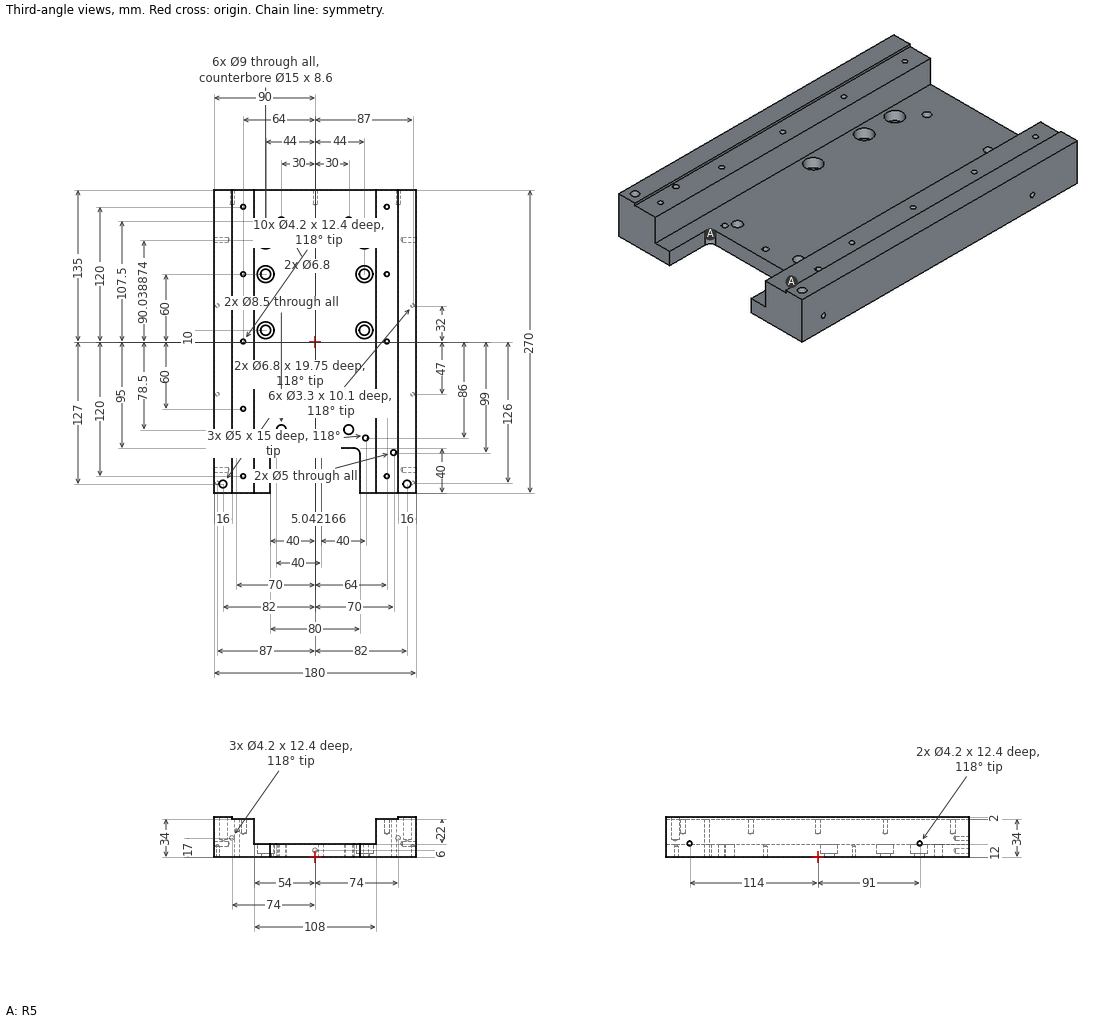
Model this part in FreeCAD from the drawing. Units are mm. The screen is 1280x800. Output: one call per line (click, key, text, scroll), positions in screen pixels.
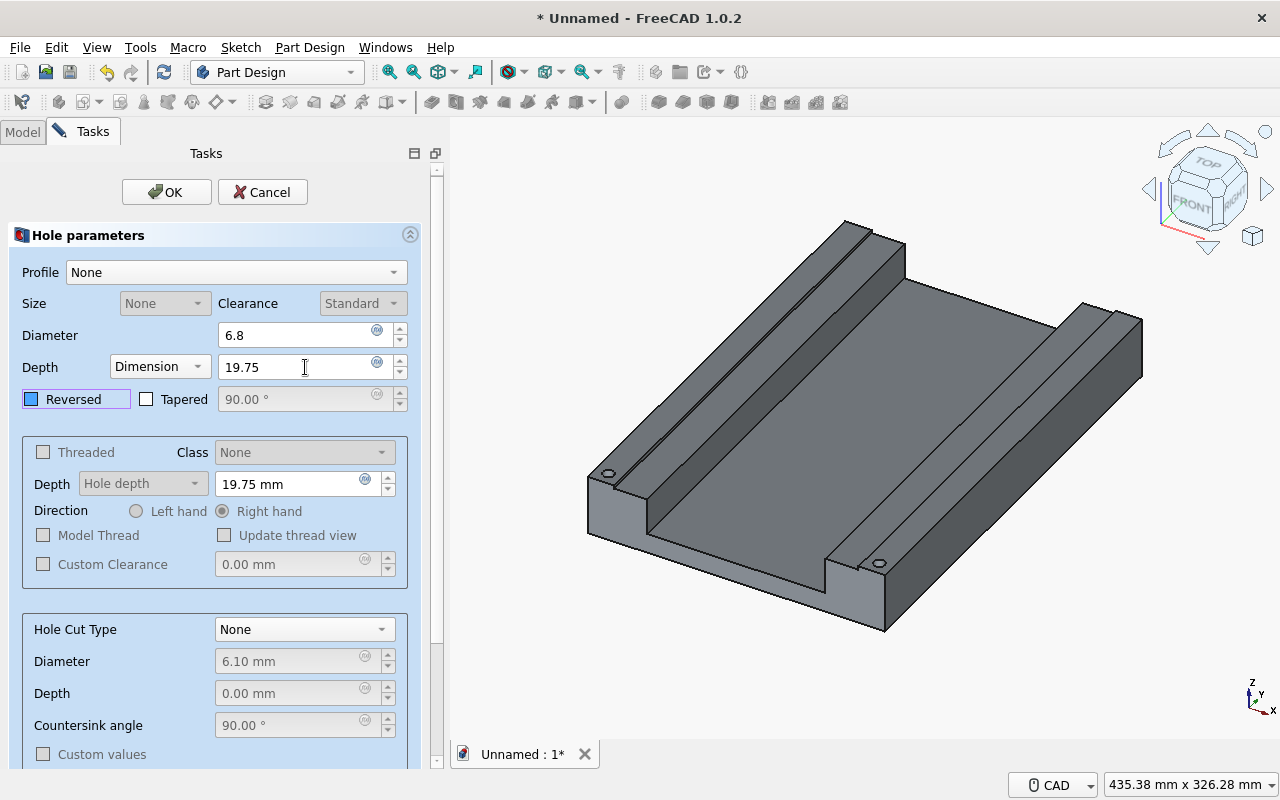
click(167, 192)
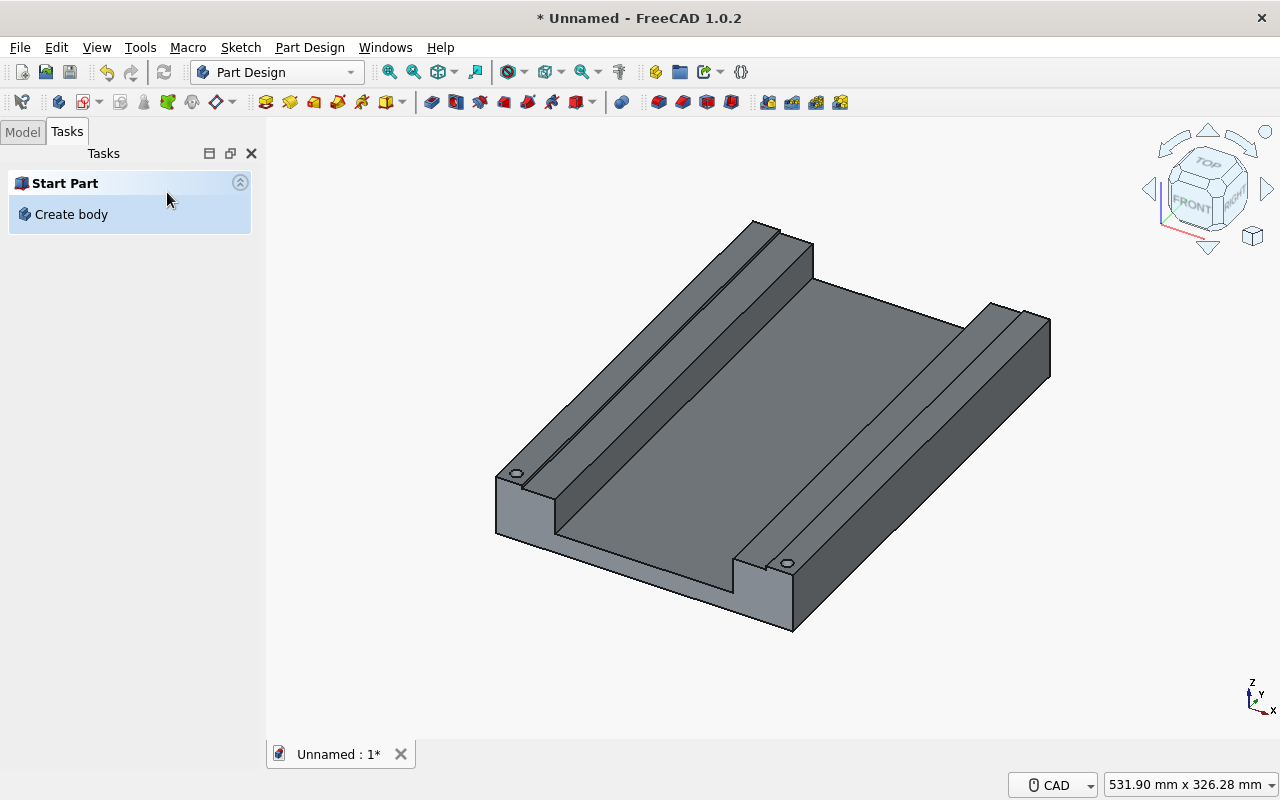
click(847, 362)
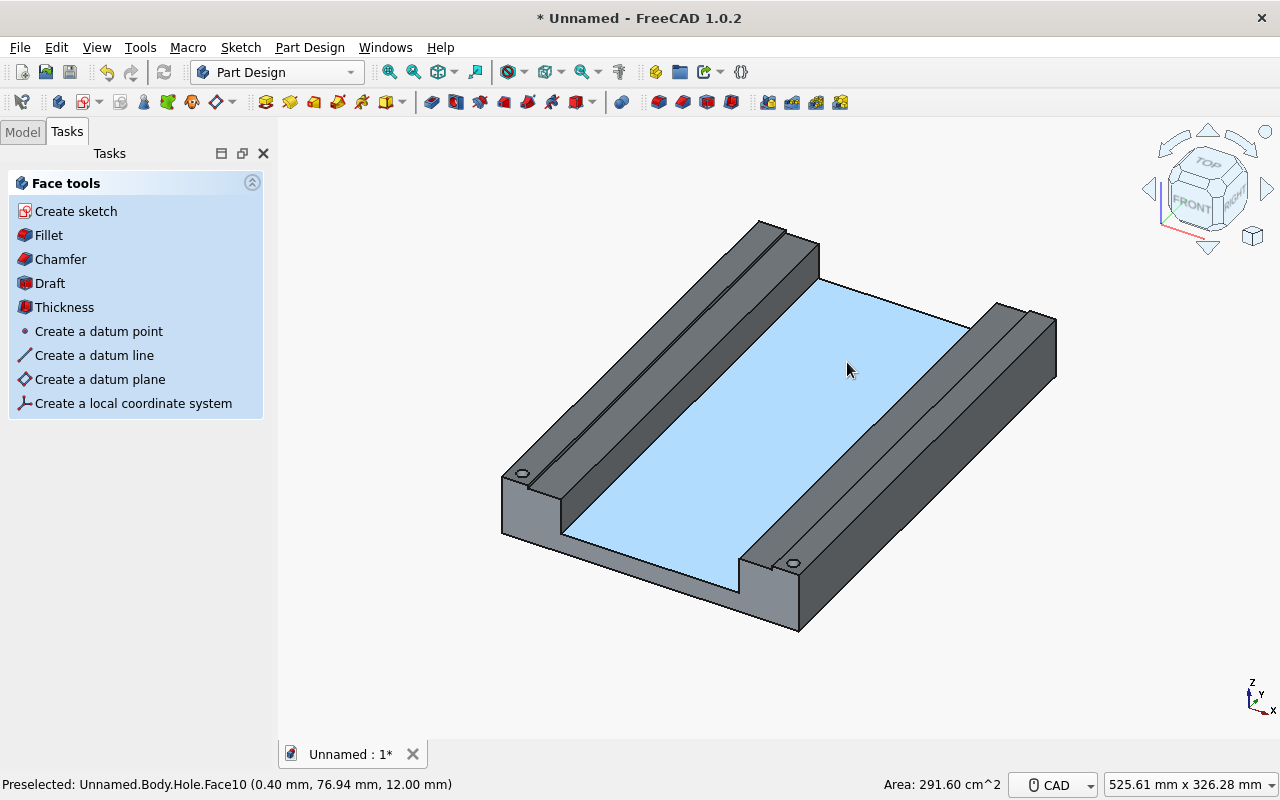
click(84, 102)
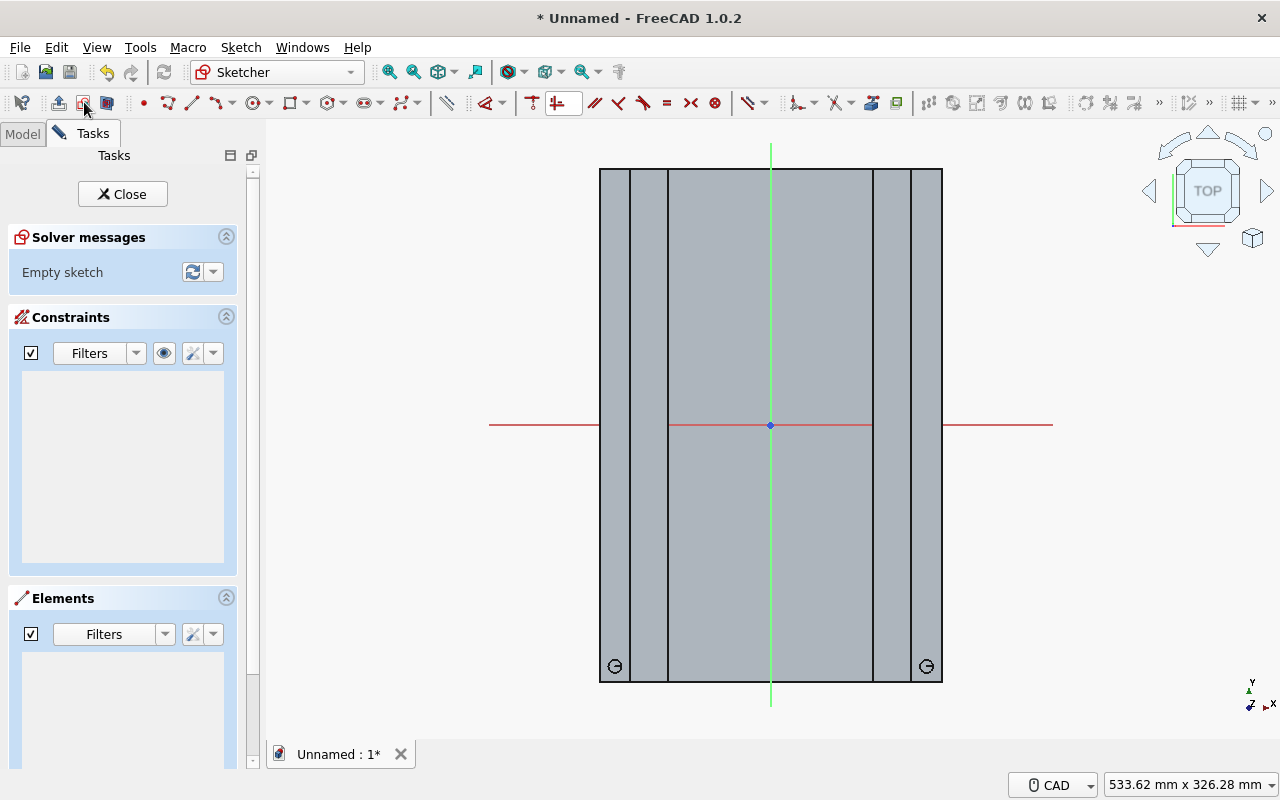
scroll(905, 711, up, 2)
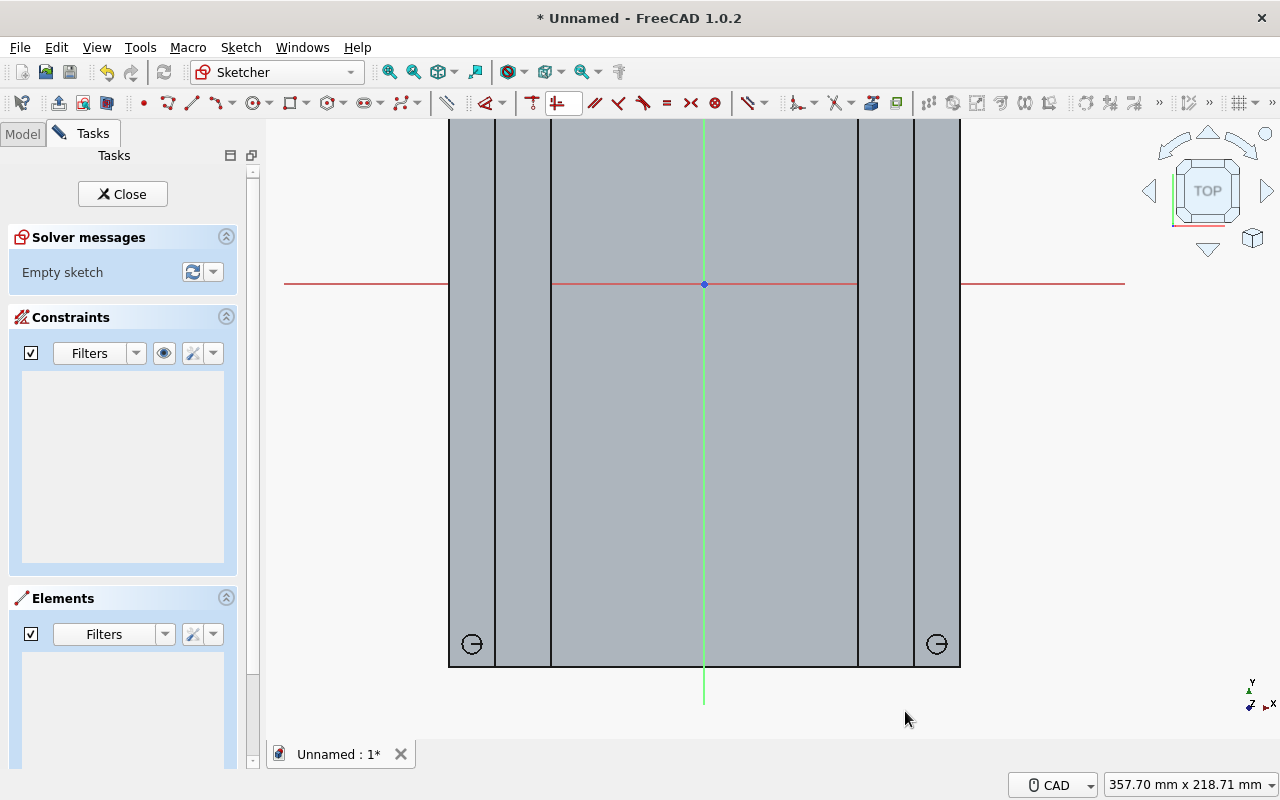
click(290, 104)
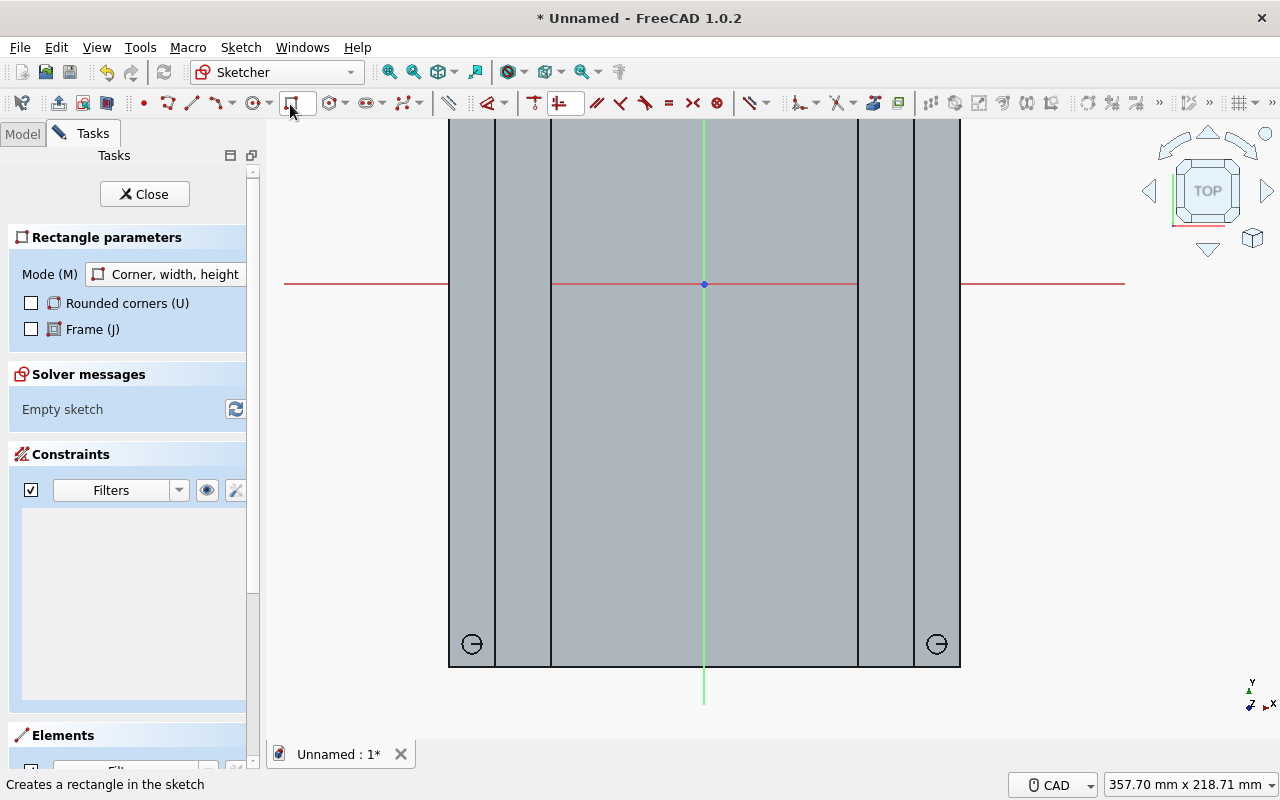
click(591, 553)
move(818, 667)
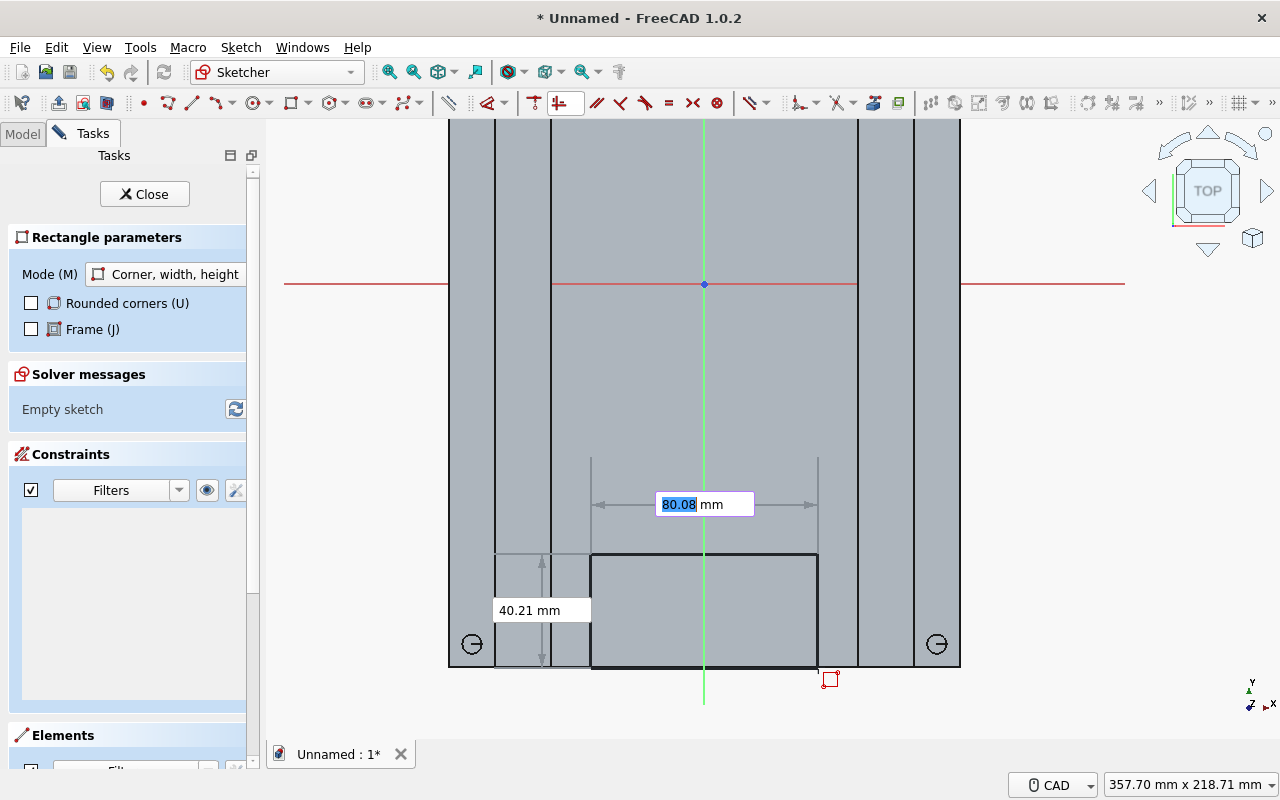
text(80)
key(Tab)
text(40)
key(Return)
key(Escape)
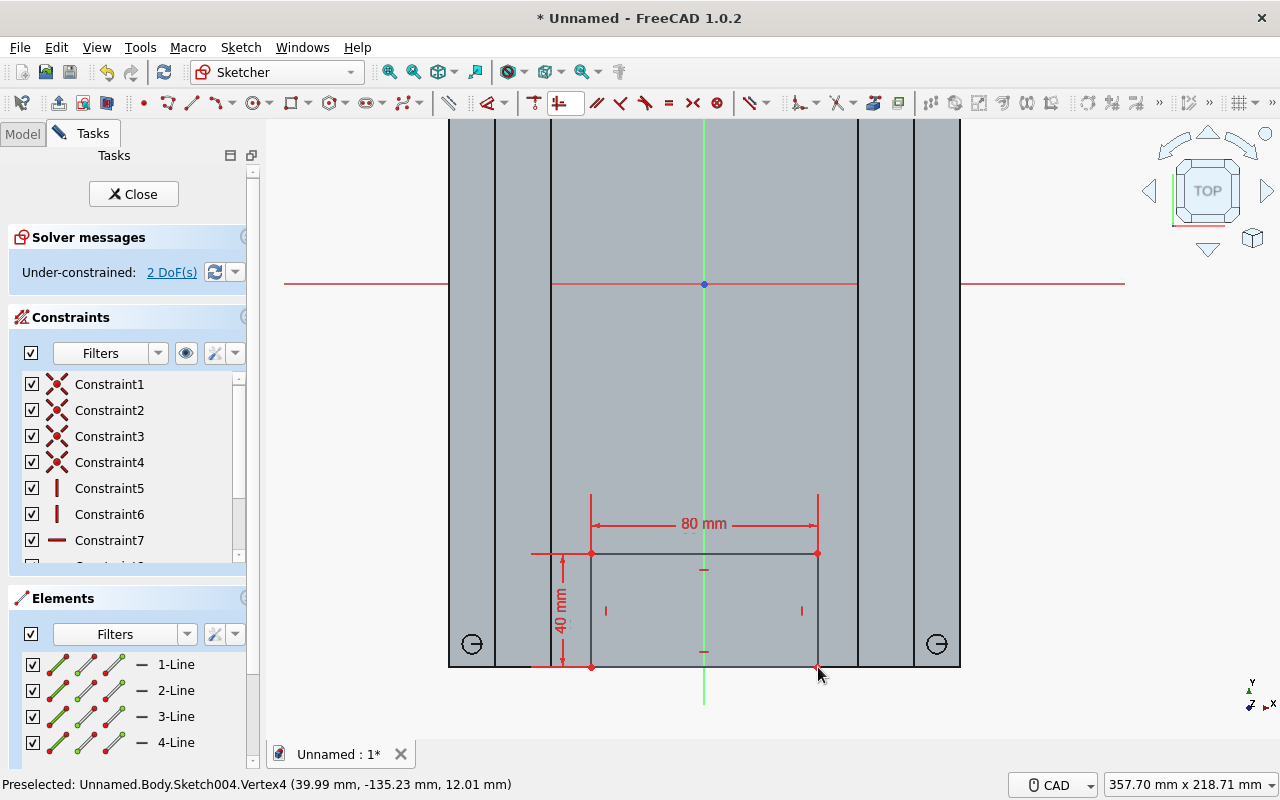
click(488, 104)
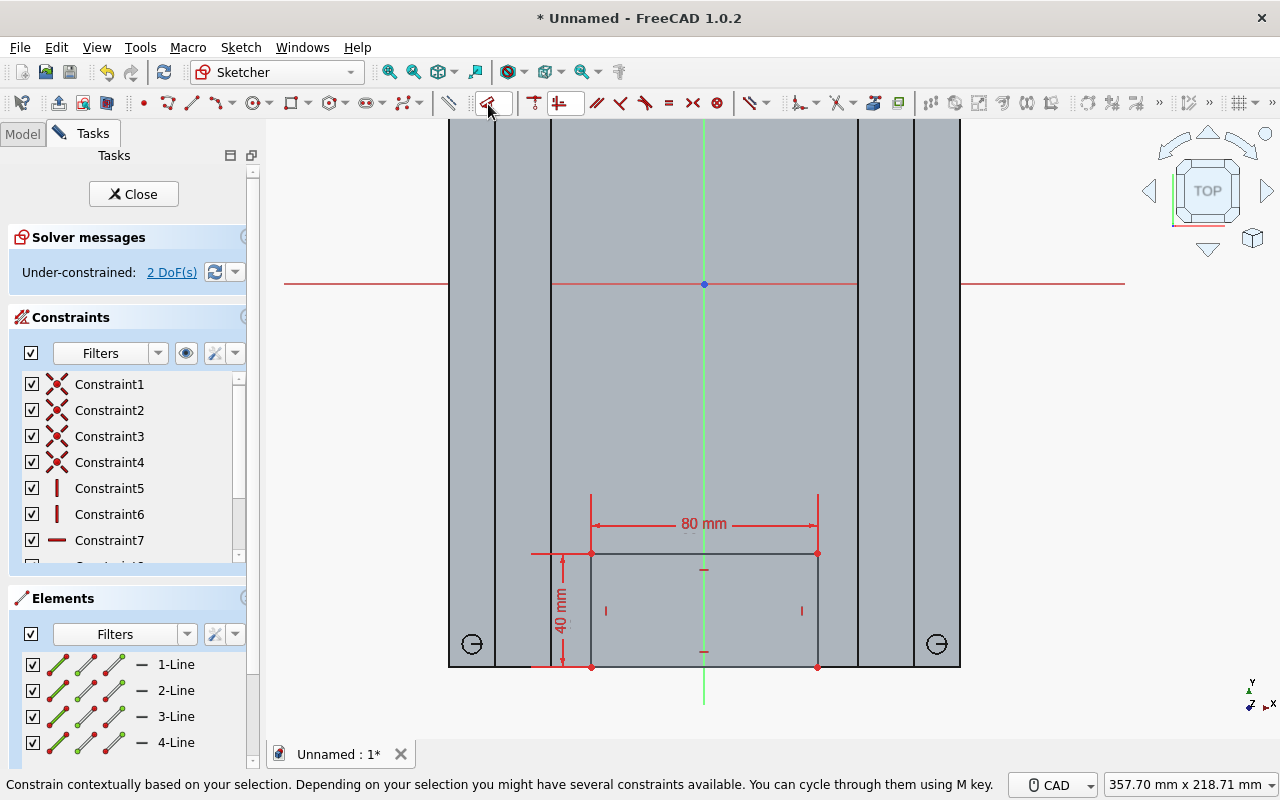
click(591, 554)
click(648, 250)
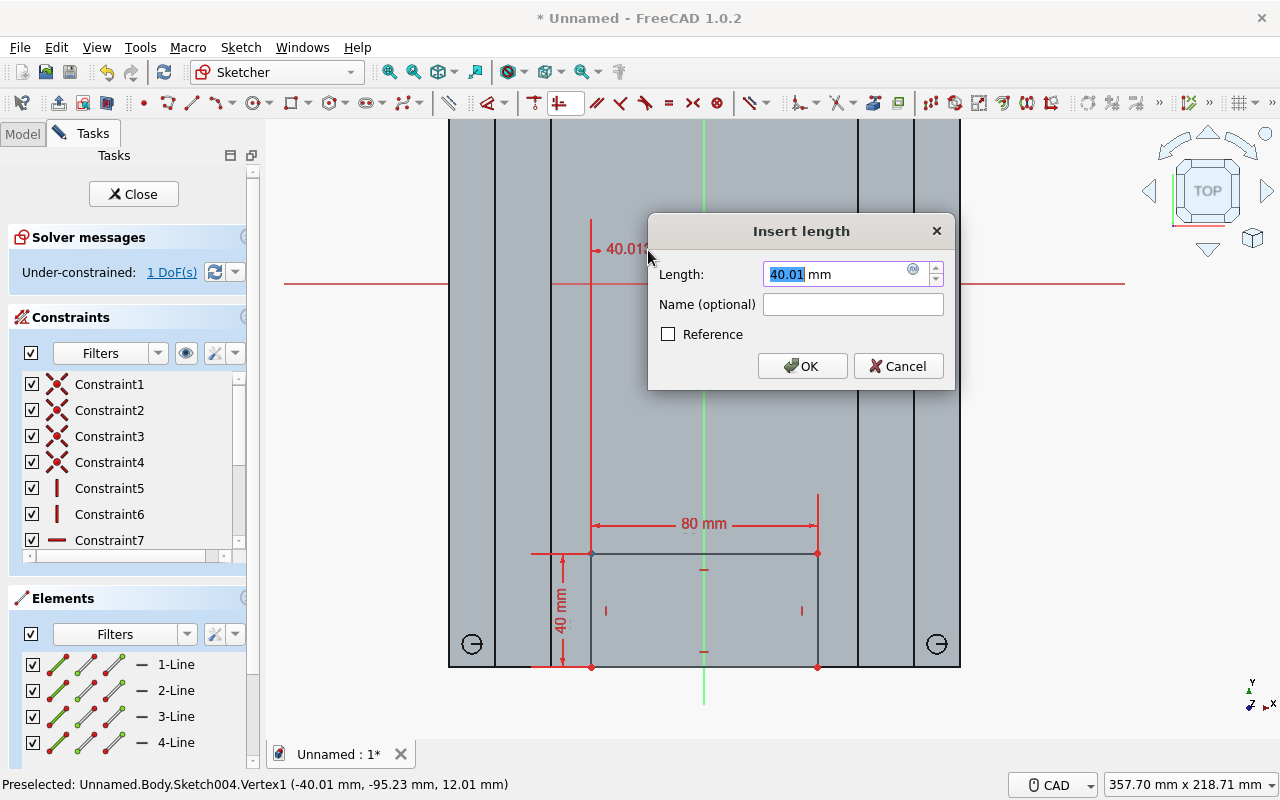
text(40)
key(Return)